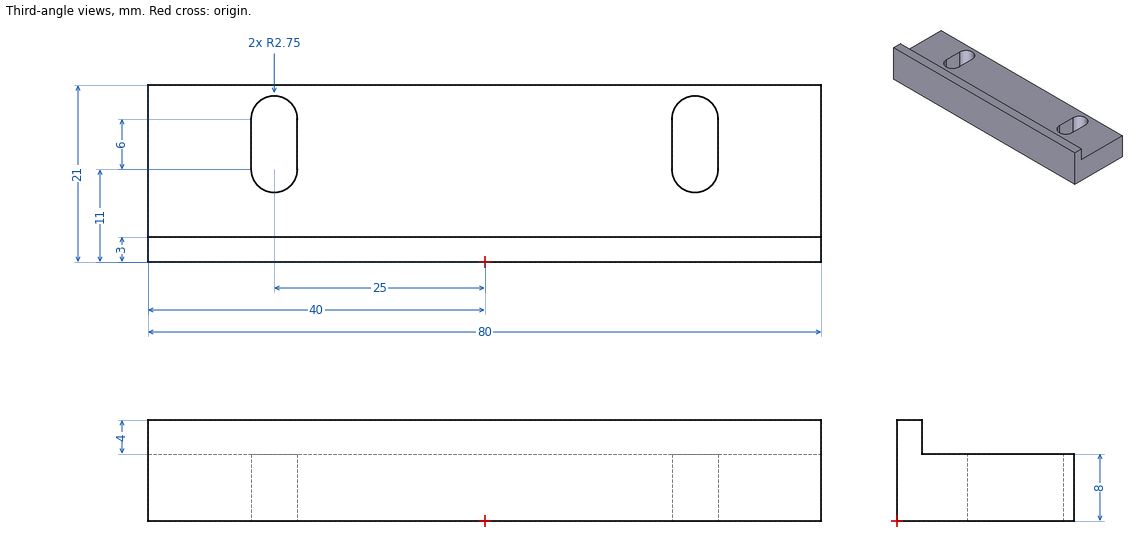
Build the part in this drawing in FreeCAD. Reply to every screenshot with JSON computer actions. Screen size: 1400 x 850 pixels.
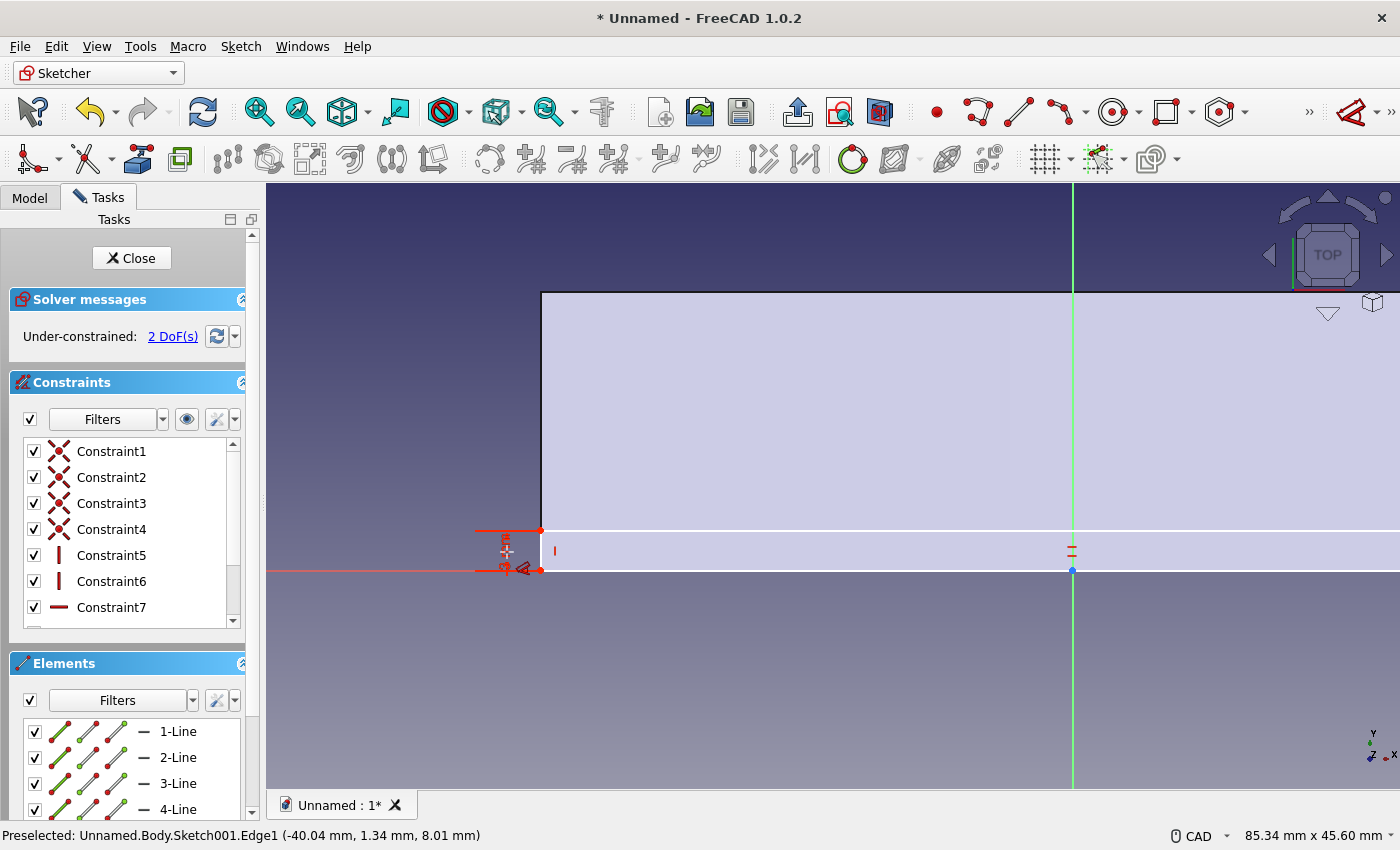
{"action": "left_click", "coordinate": [860, 571]}
{"action": "left_click", "coordinate": [888, 605]}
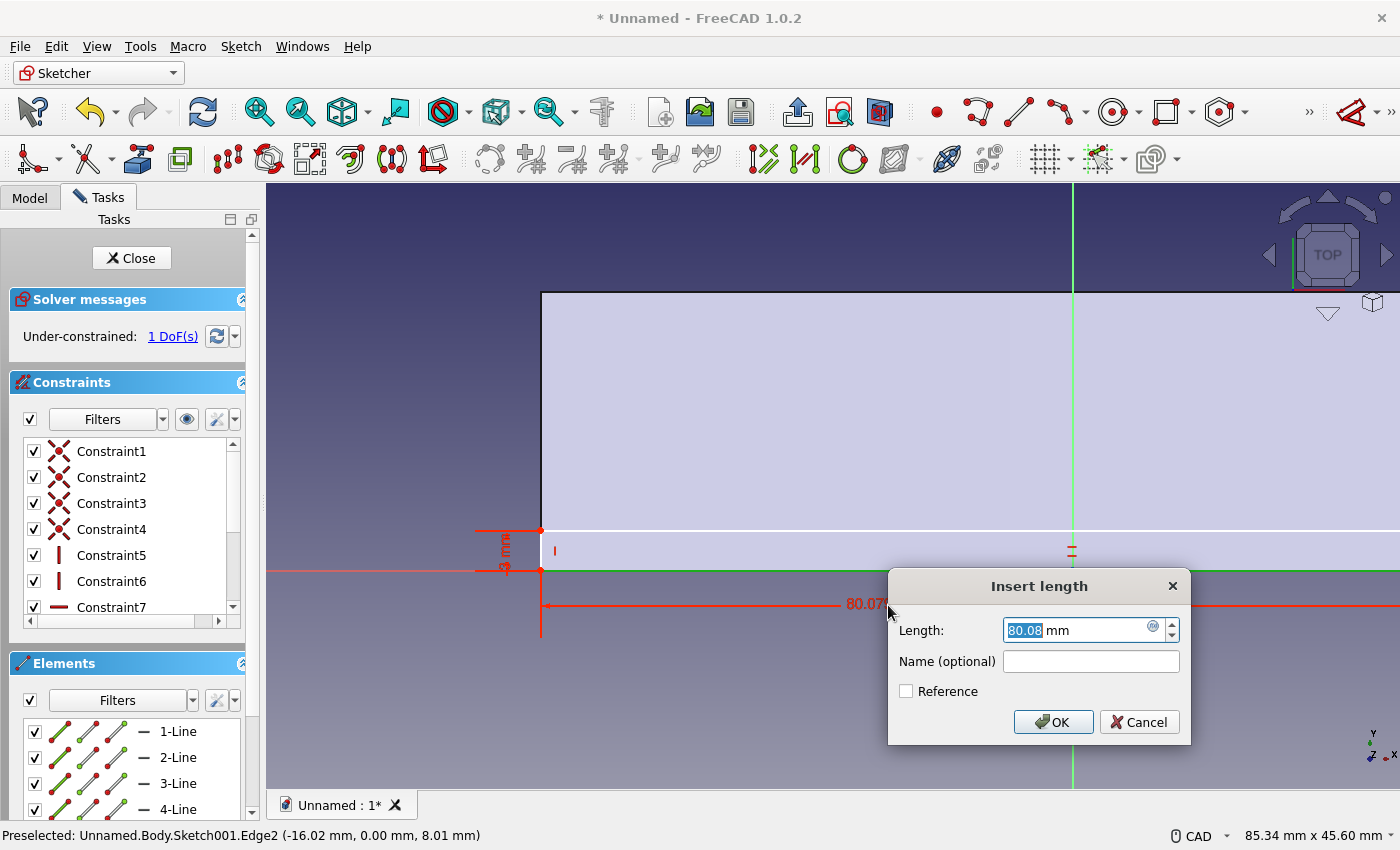
{"action": "type", "text": "80"}
{"action": "key", "text": "Return"}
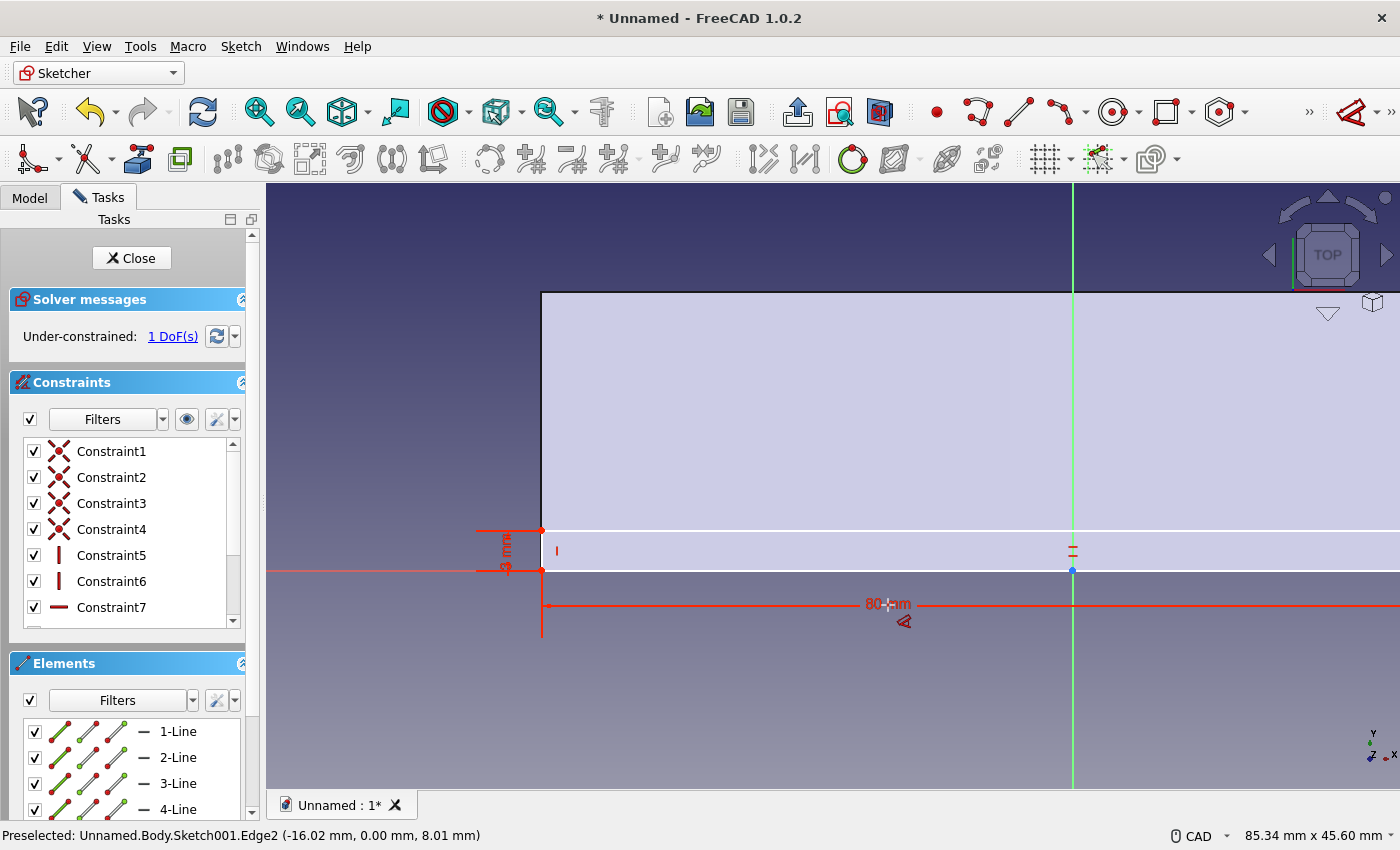
{"action": "left_click", "coordinate": [542, 531]}
{"action": "left_click", "coordinate": [807, 605]}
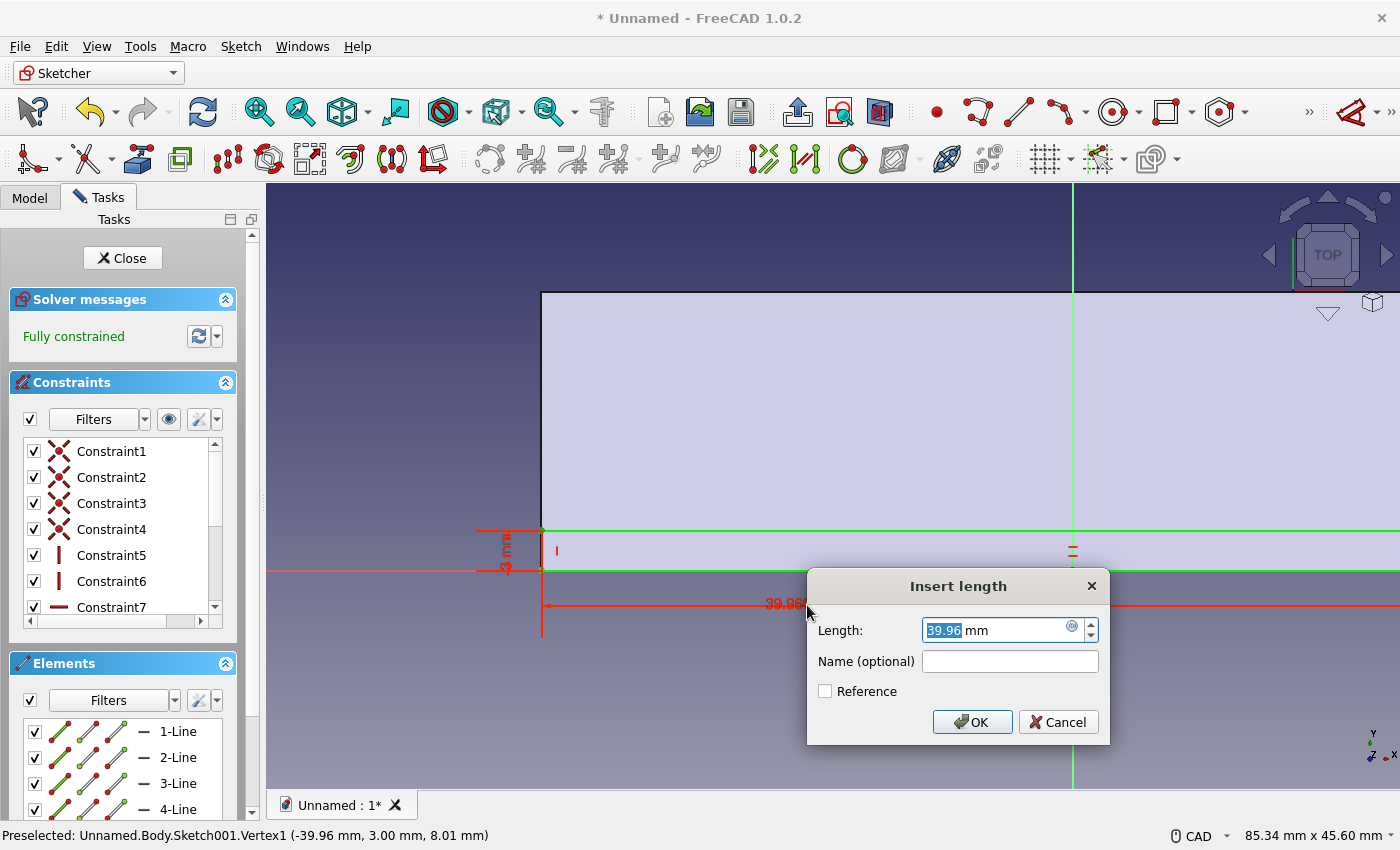
{"action": "type", "text": "40"}
{"action": "key", "text": "Return"}
{"action": "key", "text": "Escape"}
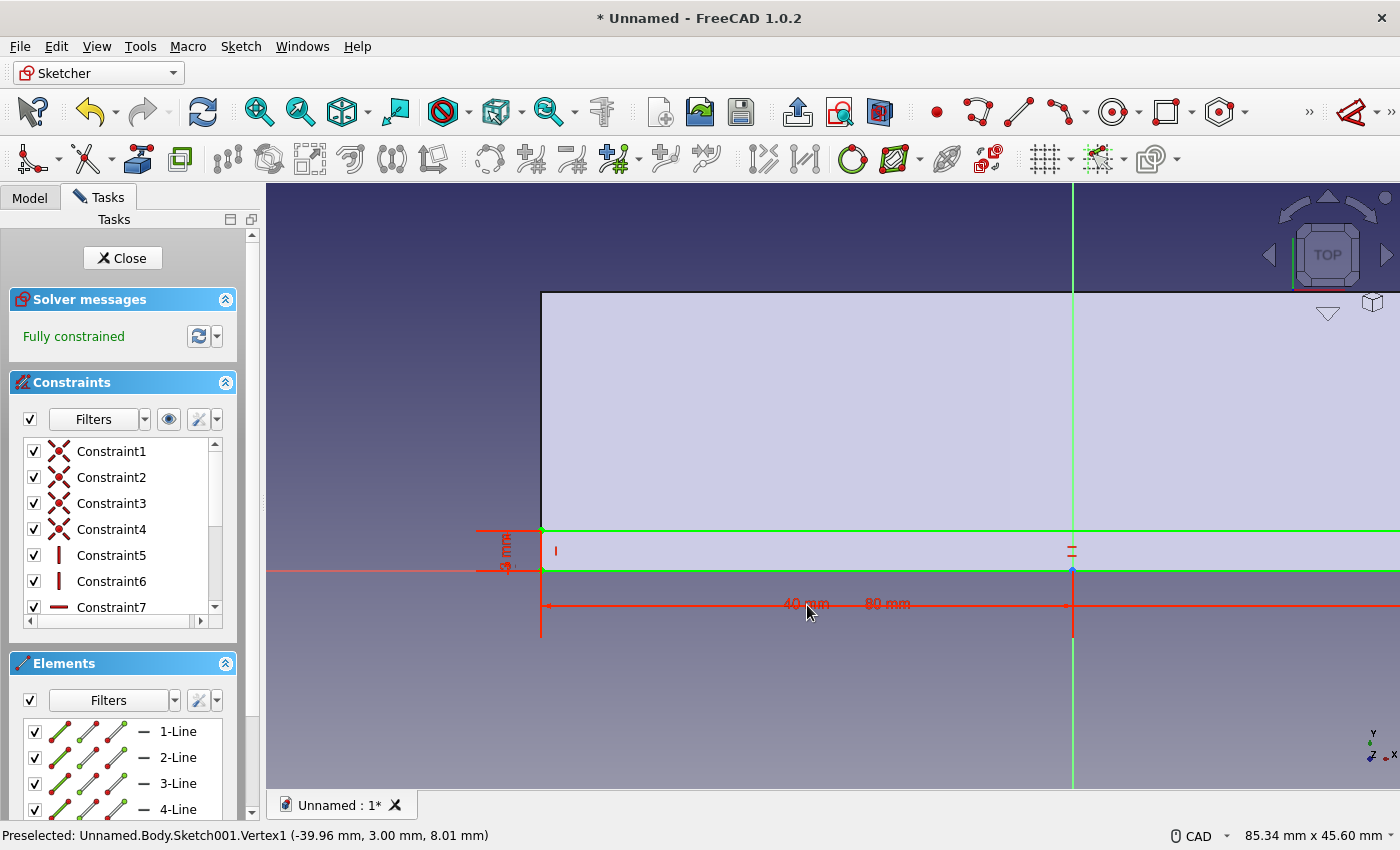
{"action": "left_click", "coordinate": [123, 258]}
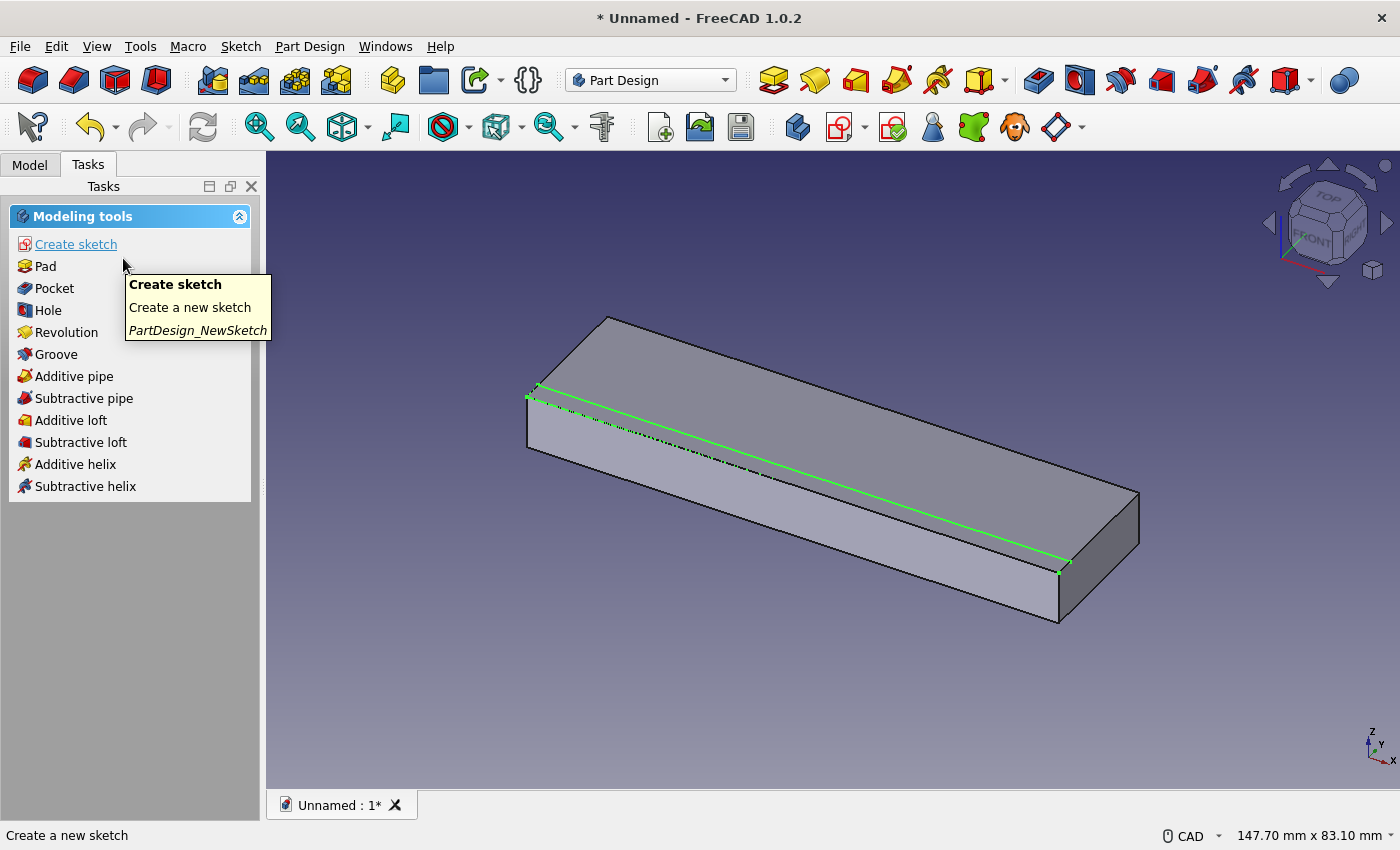
{"action": "left_click", "coordinate": [774, 80]}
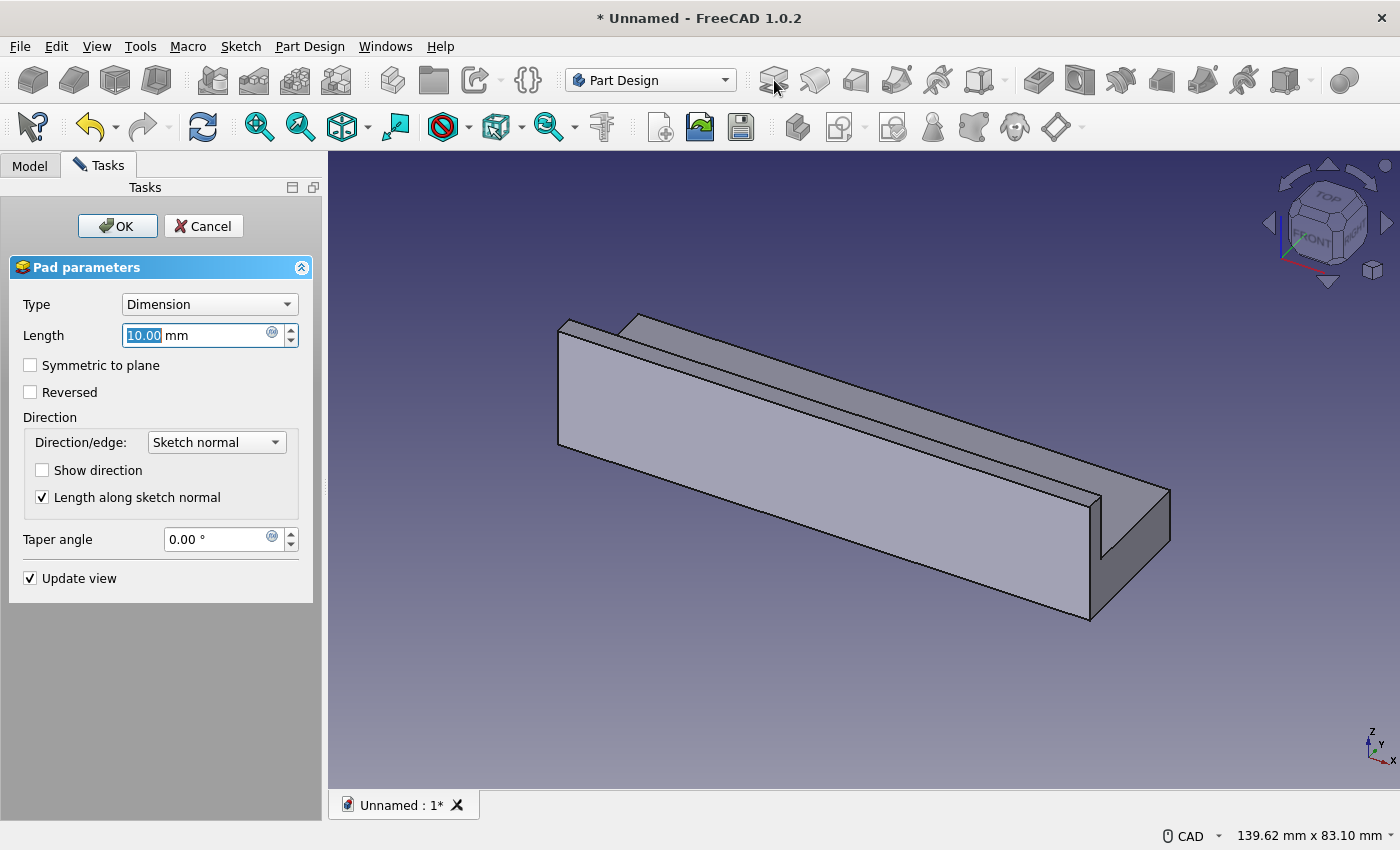
{"action": "type", "text": "4"}
{"action": "key", "text": "Tab"}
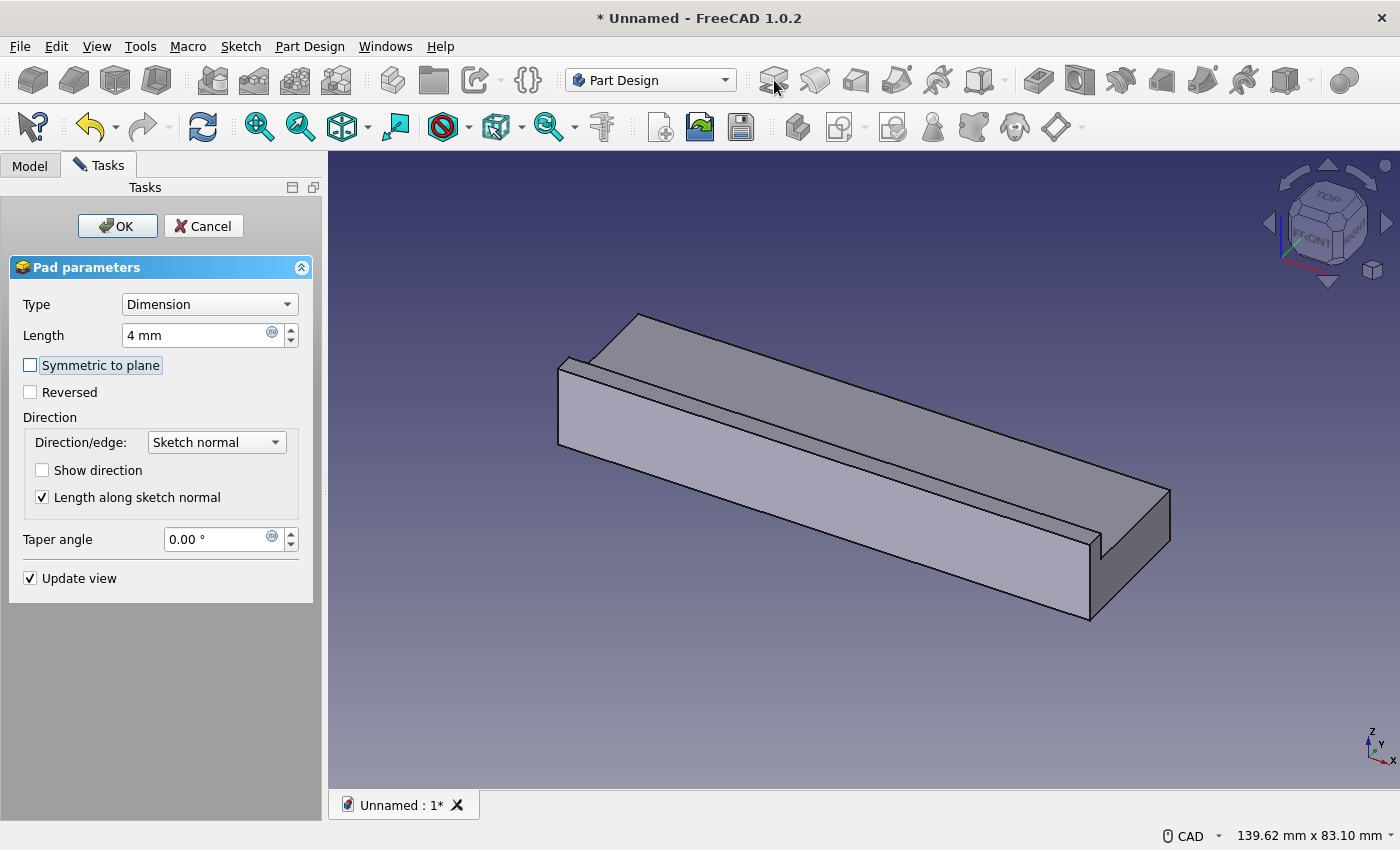
{"action": "left_click", "coordinate": [118, 226]}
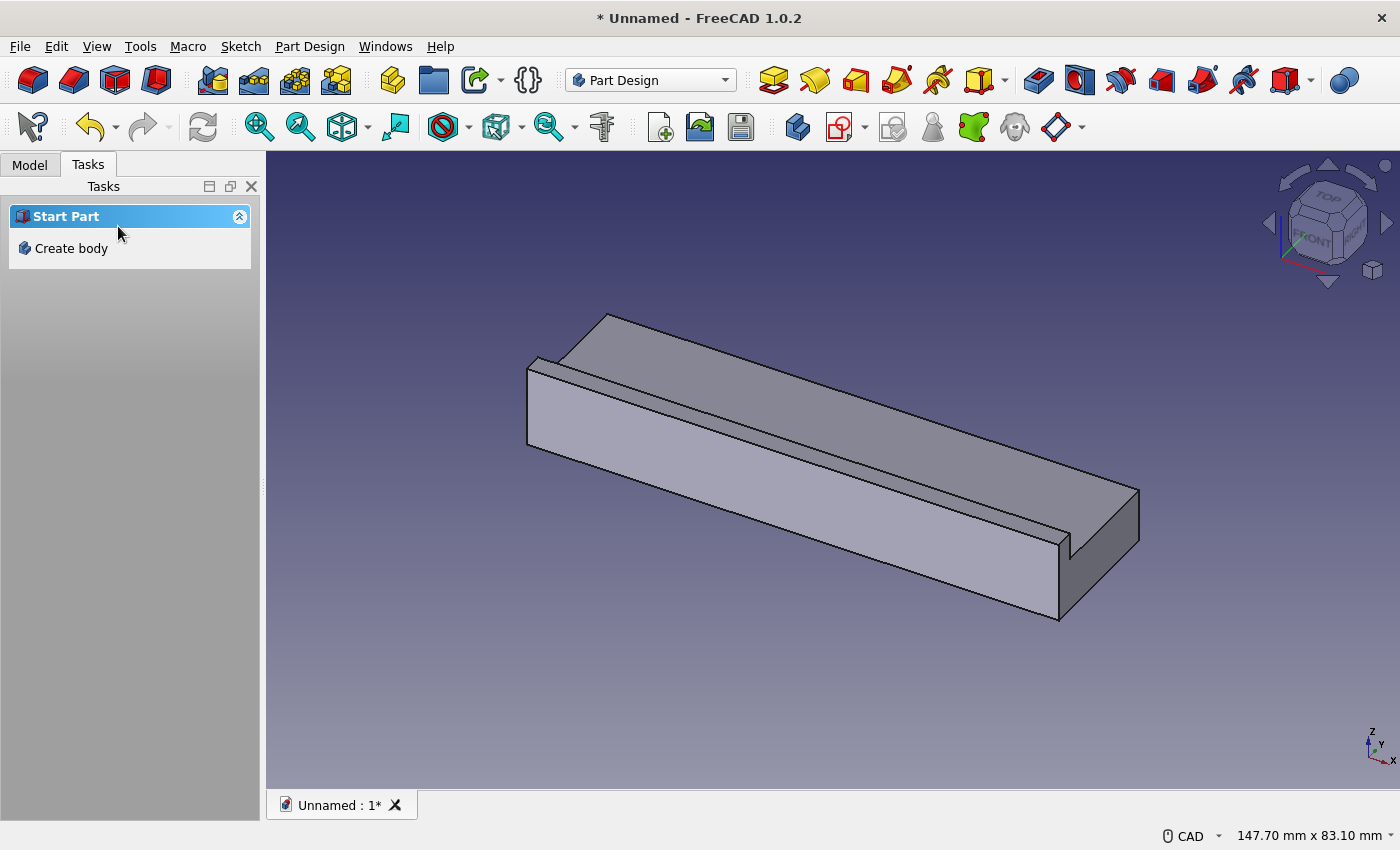
{"action": "left_click", "coordinate": [991, 486]}